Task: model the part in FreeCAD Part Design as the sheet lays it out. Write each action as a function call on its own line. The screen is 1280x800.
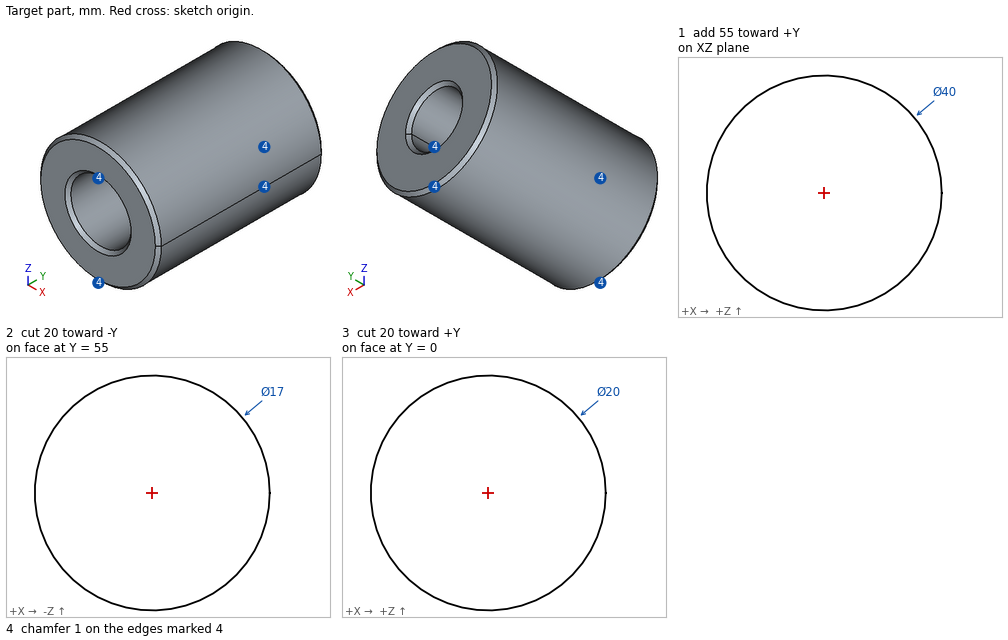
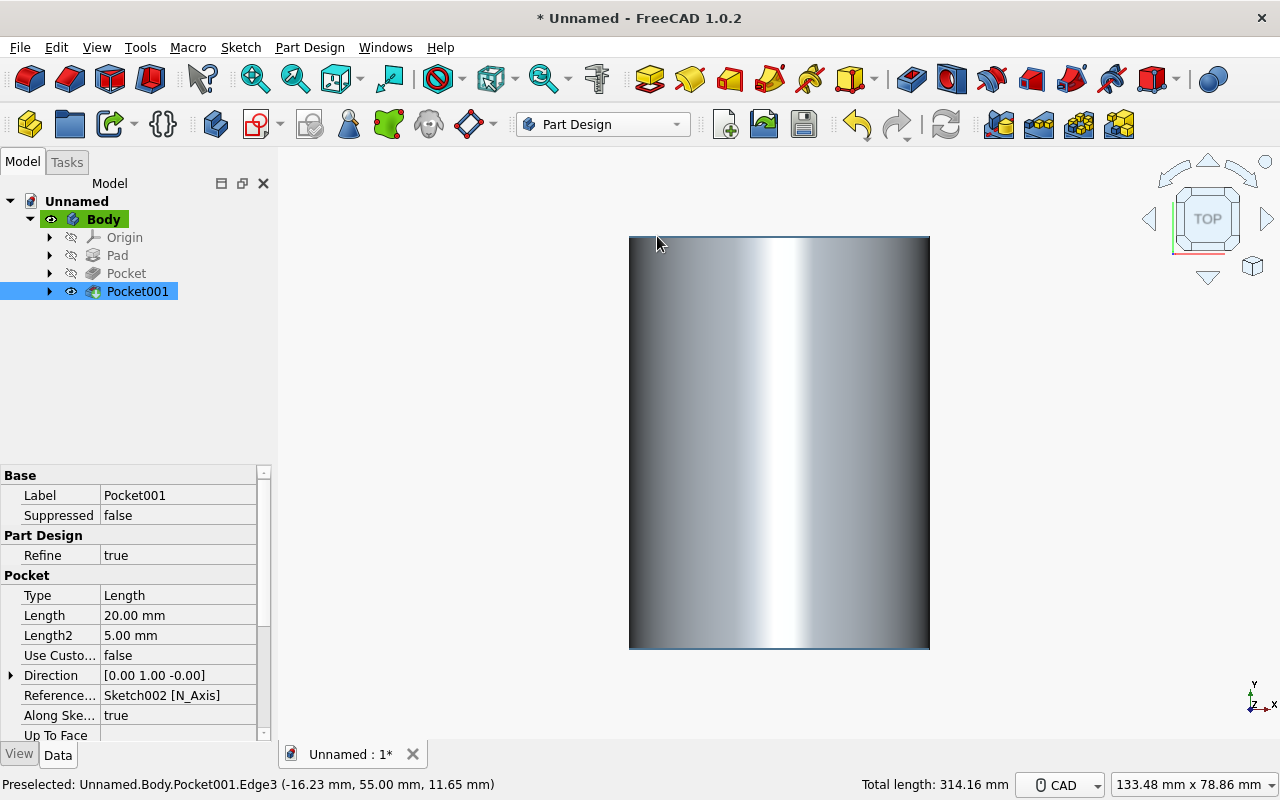
key(0)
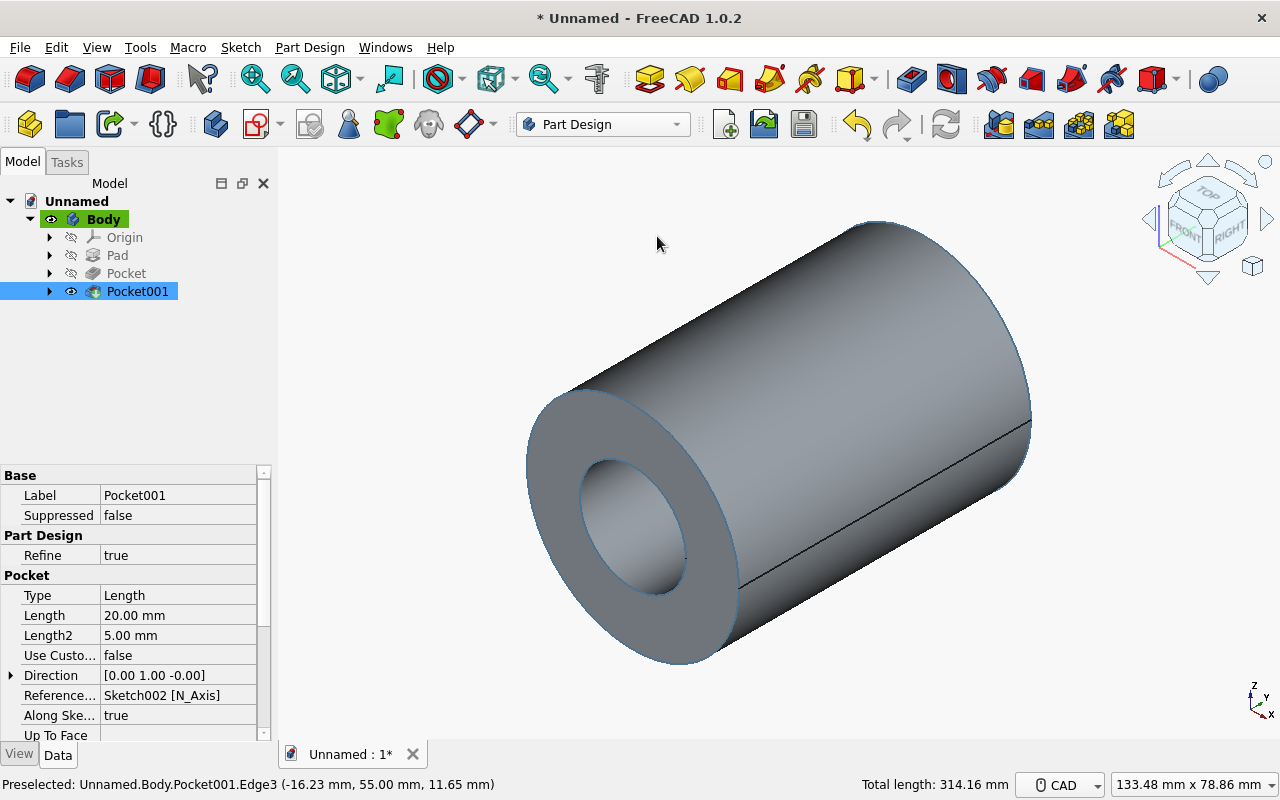
key(1)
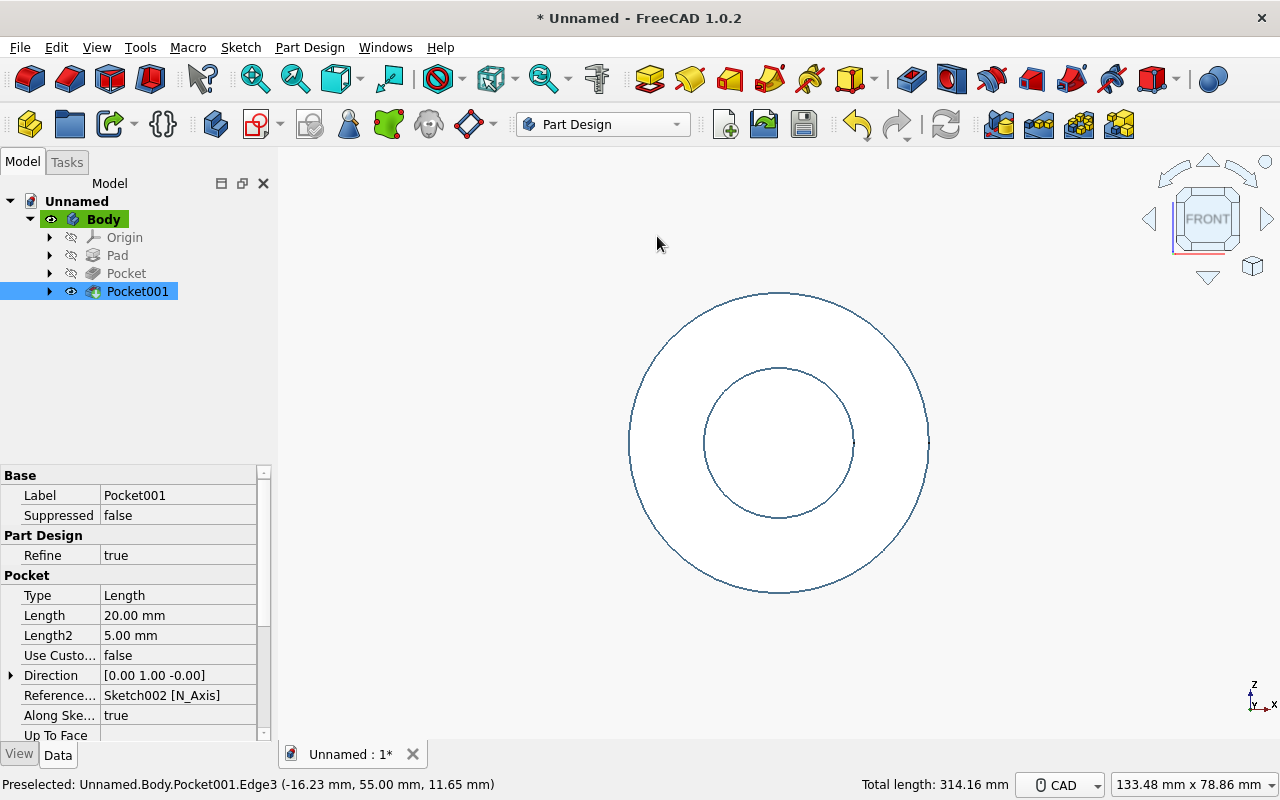
key(3)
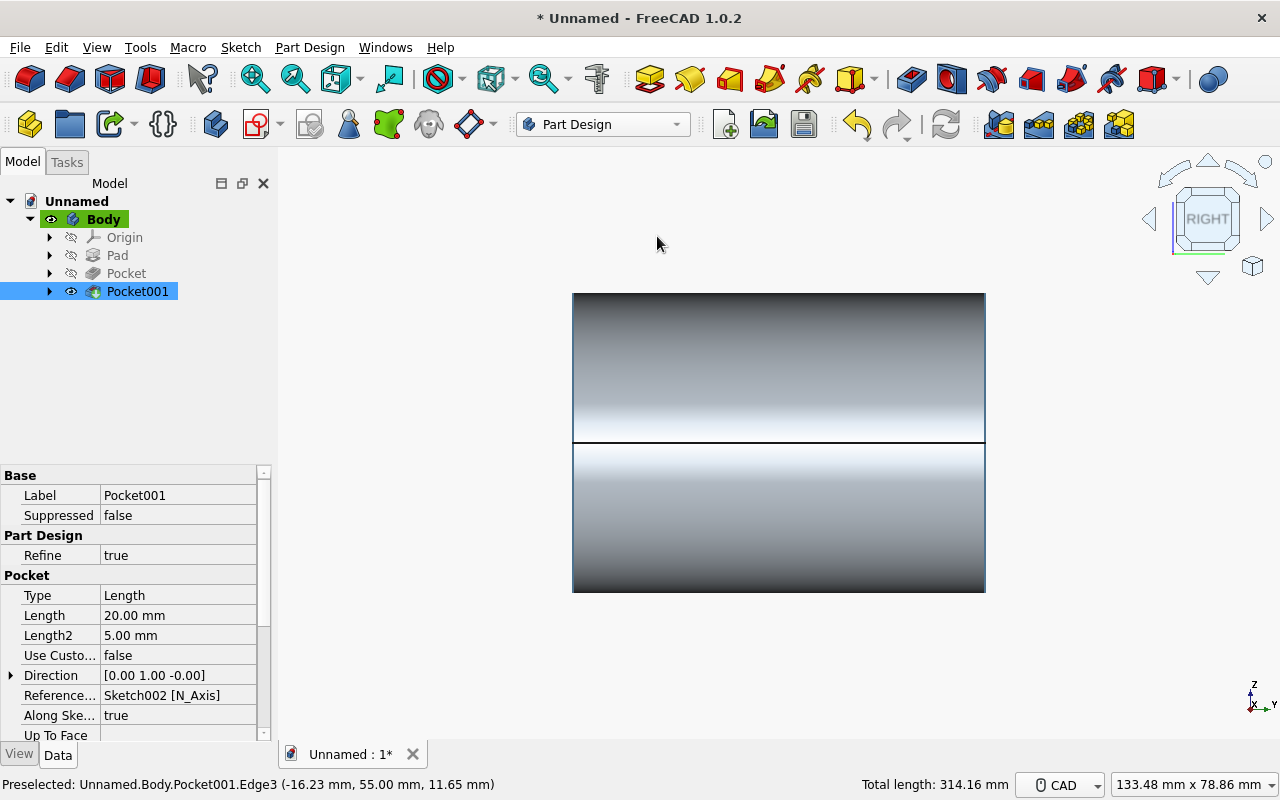
key(5)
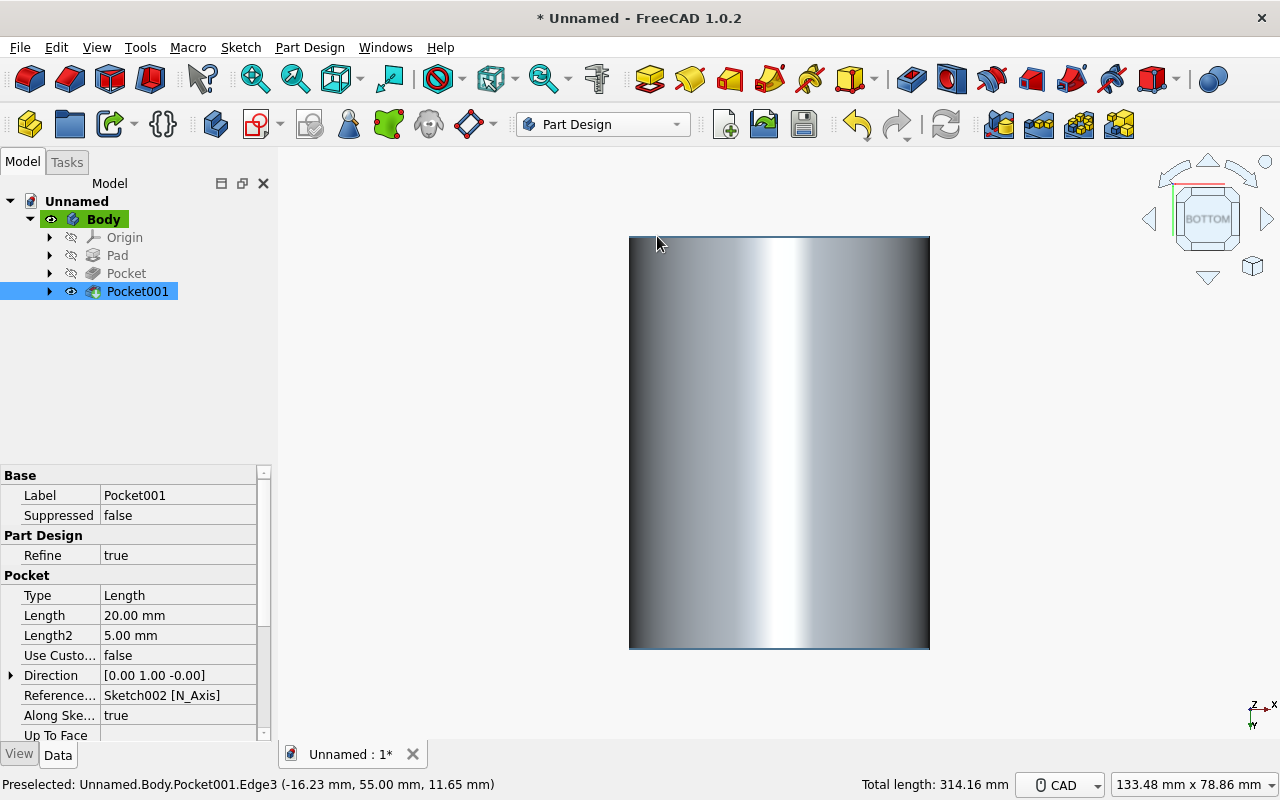
key(4)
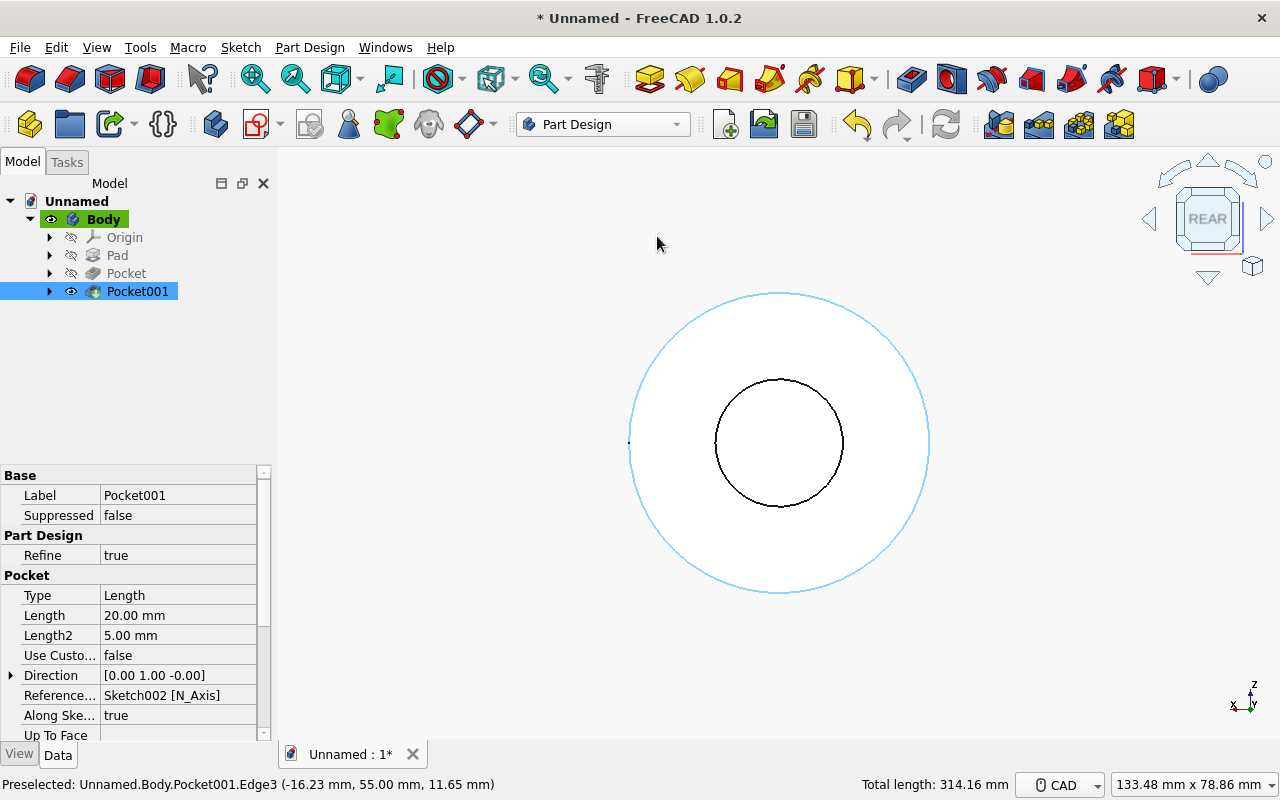
click(843, 442, ctrl)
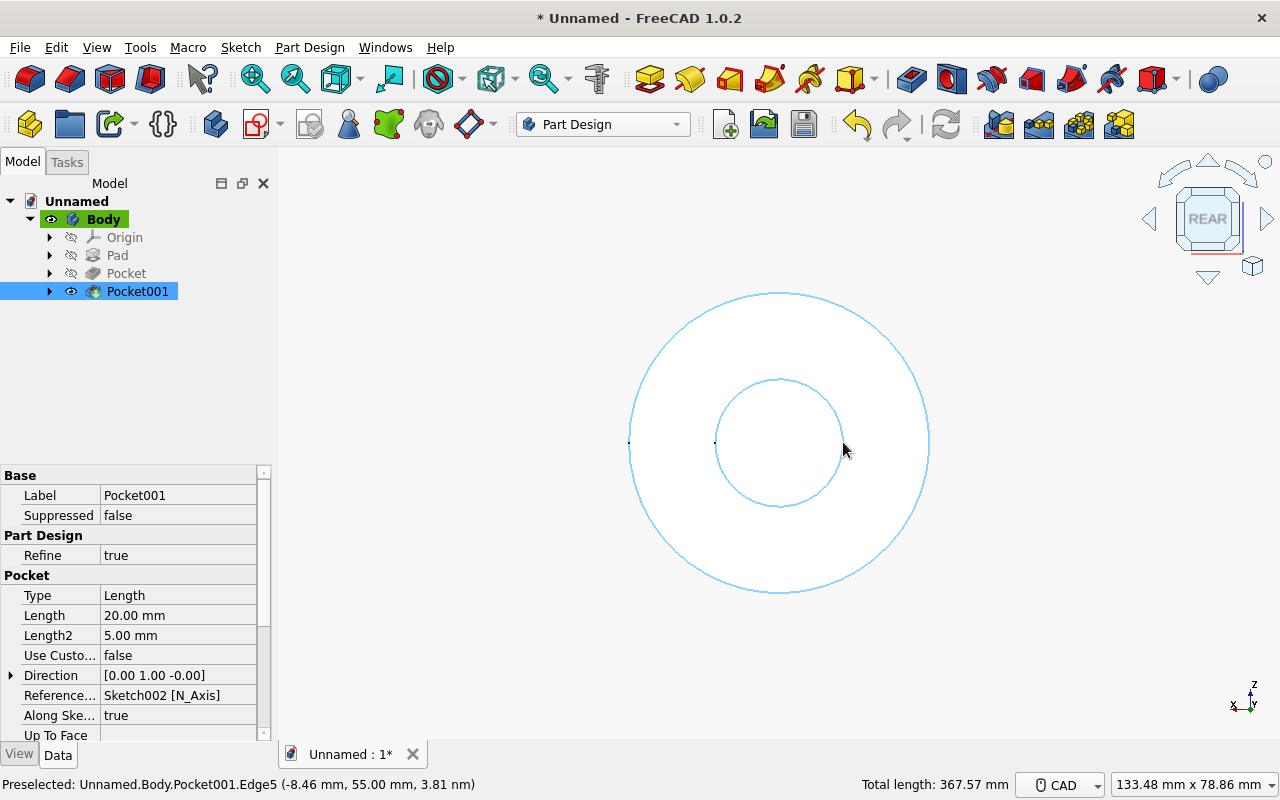
click(70, 80)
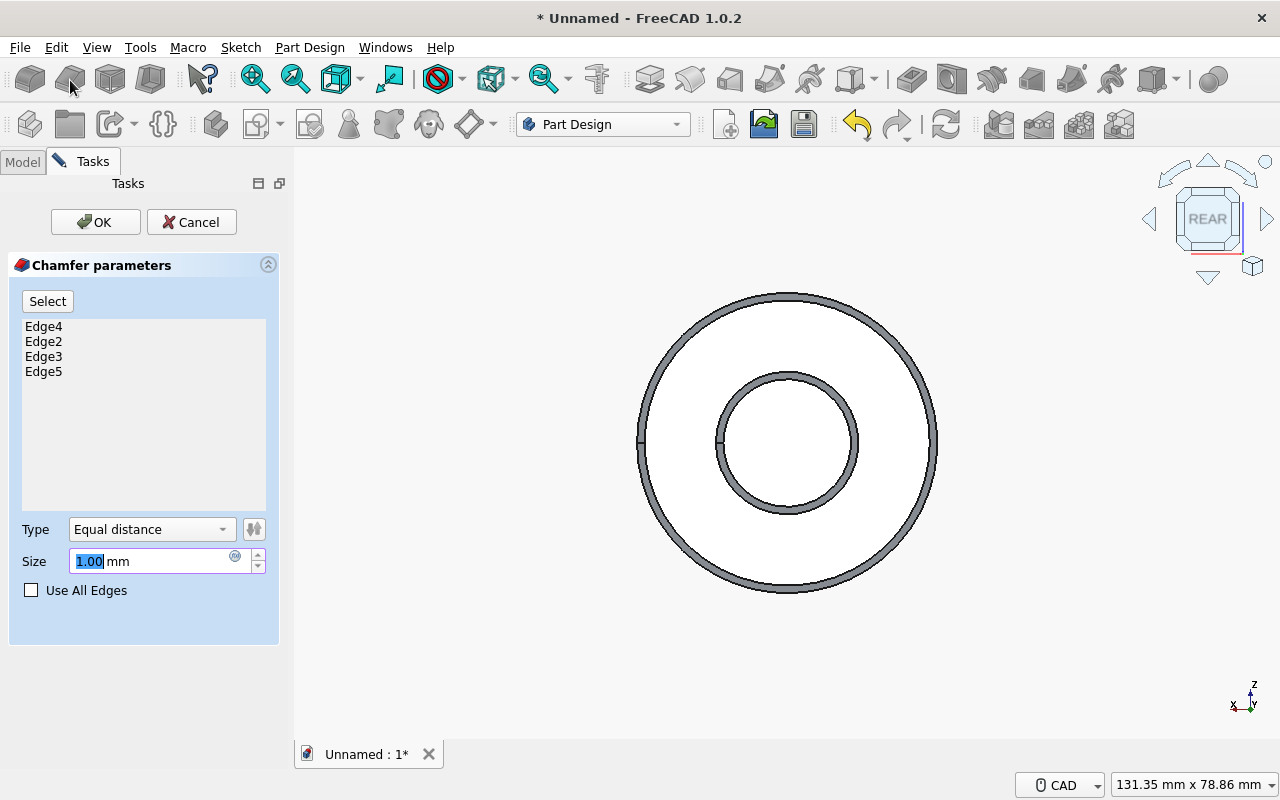
text(1)
key(Tab)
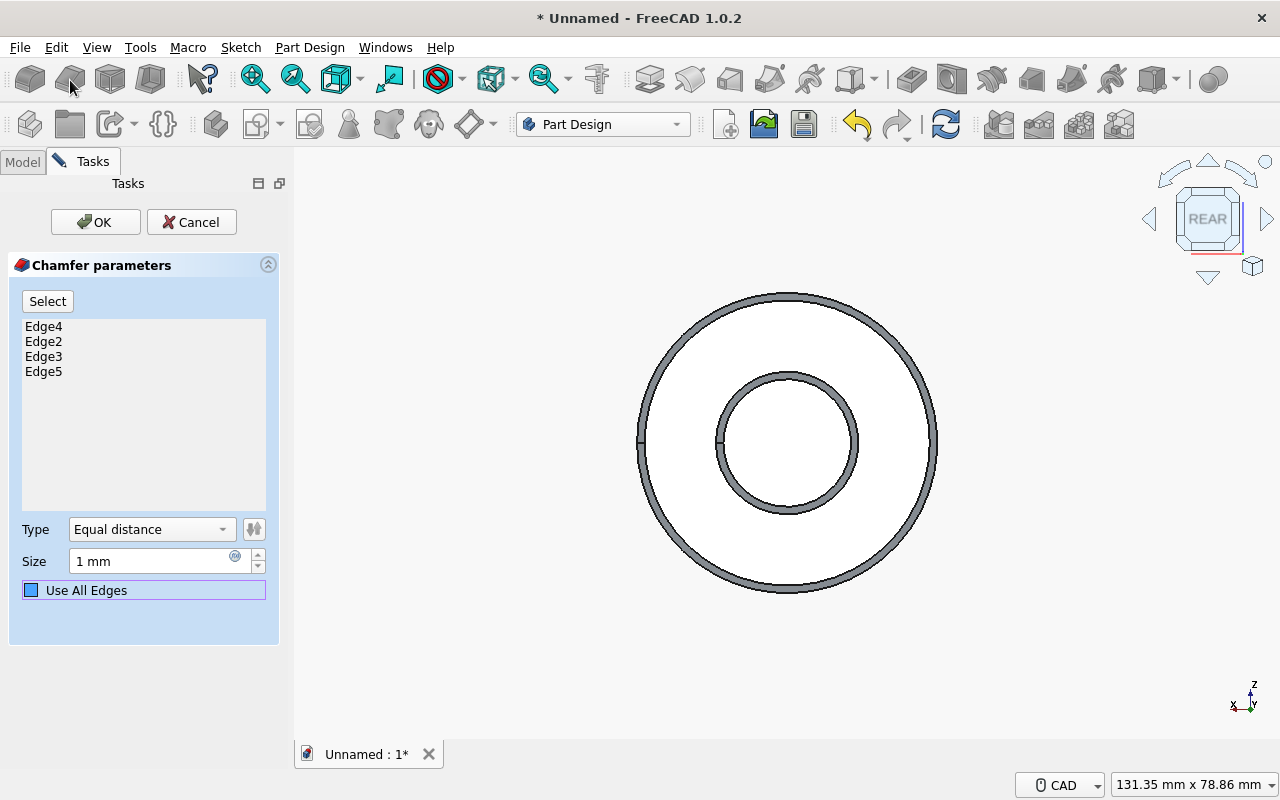
click(96, 222)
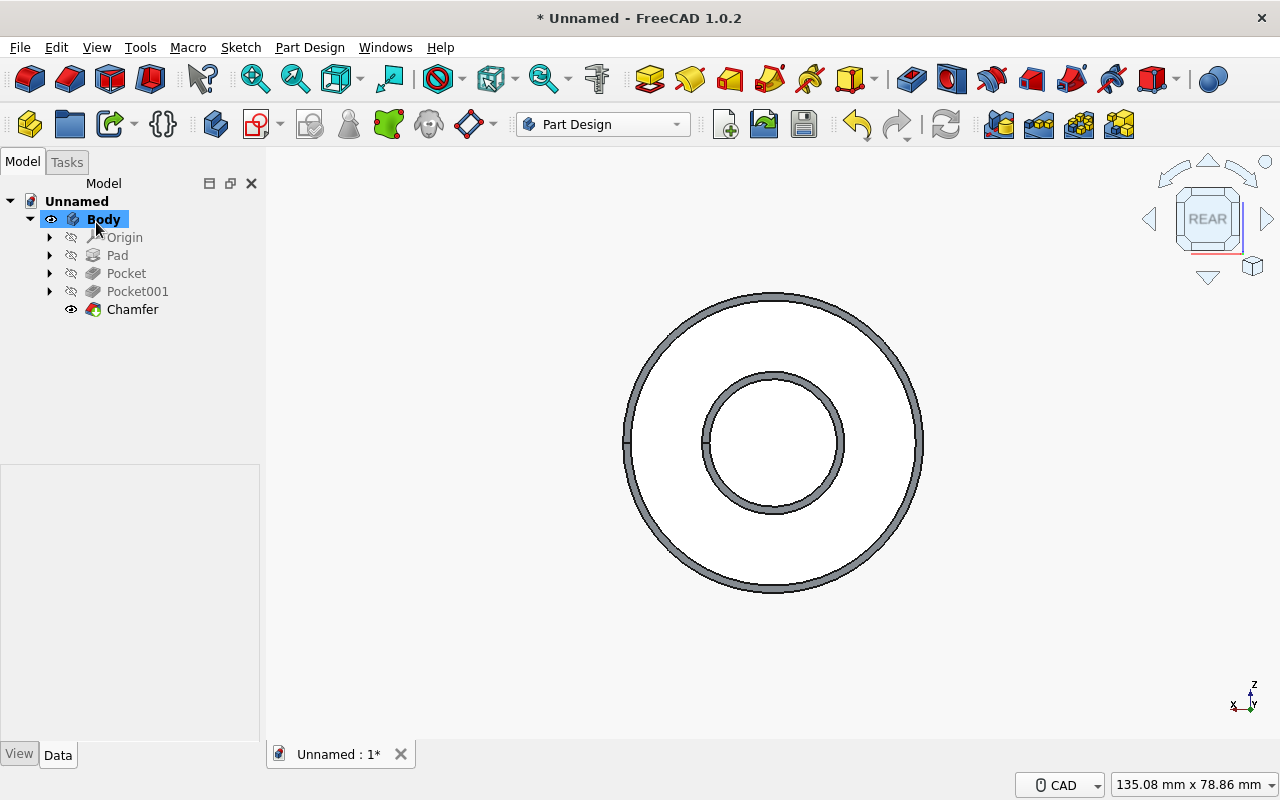
key(0)